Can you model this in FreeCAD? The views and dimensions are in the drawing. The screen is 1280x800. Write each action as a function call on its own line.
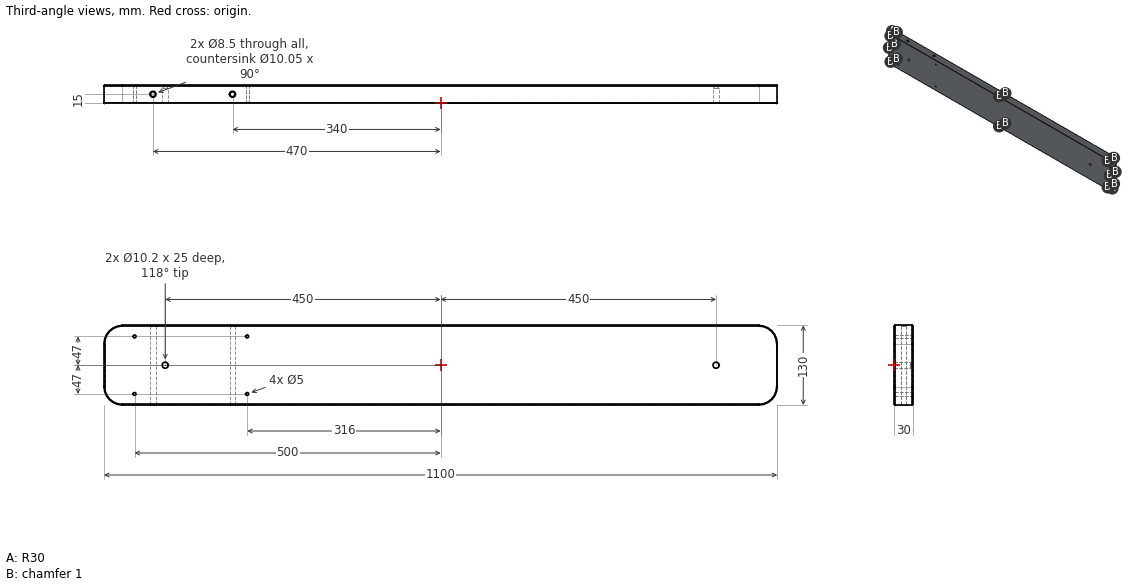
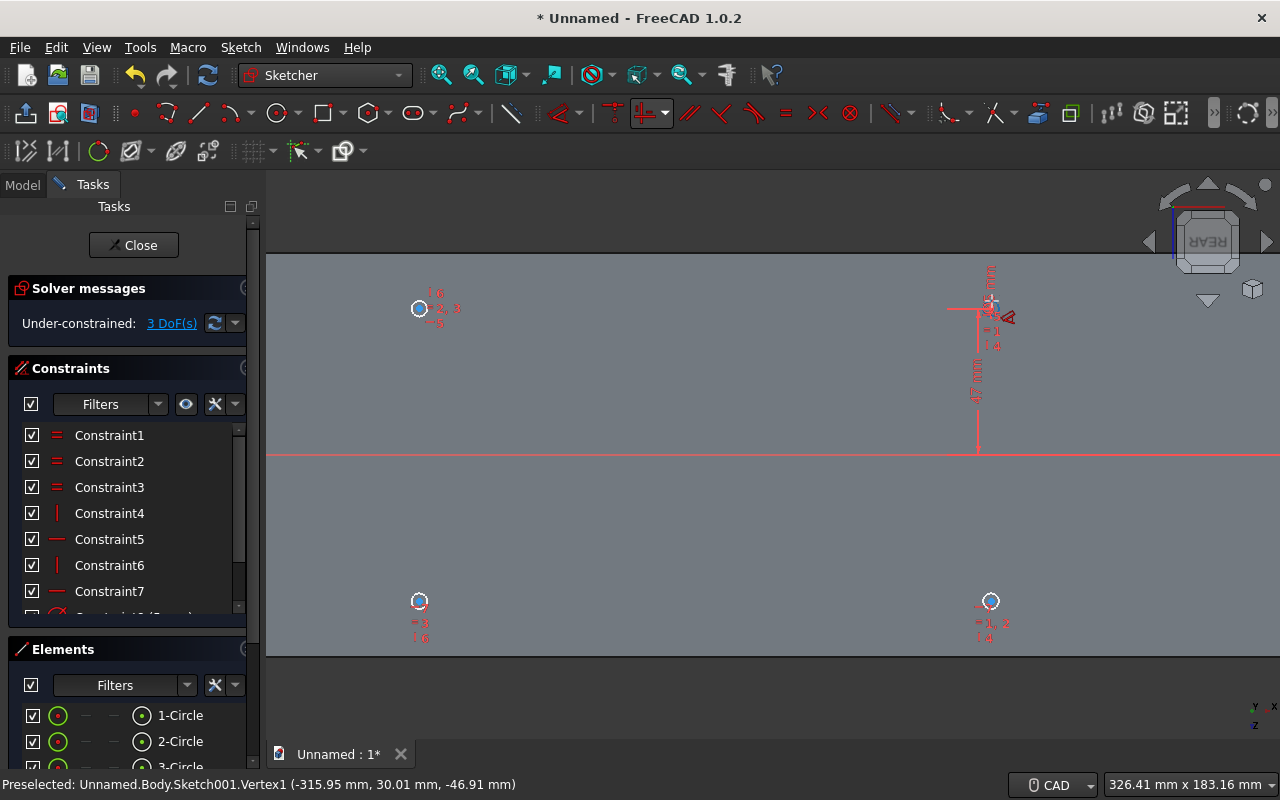
click(991, 601)
click(957, 528)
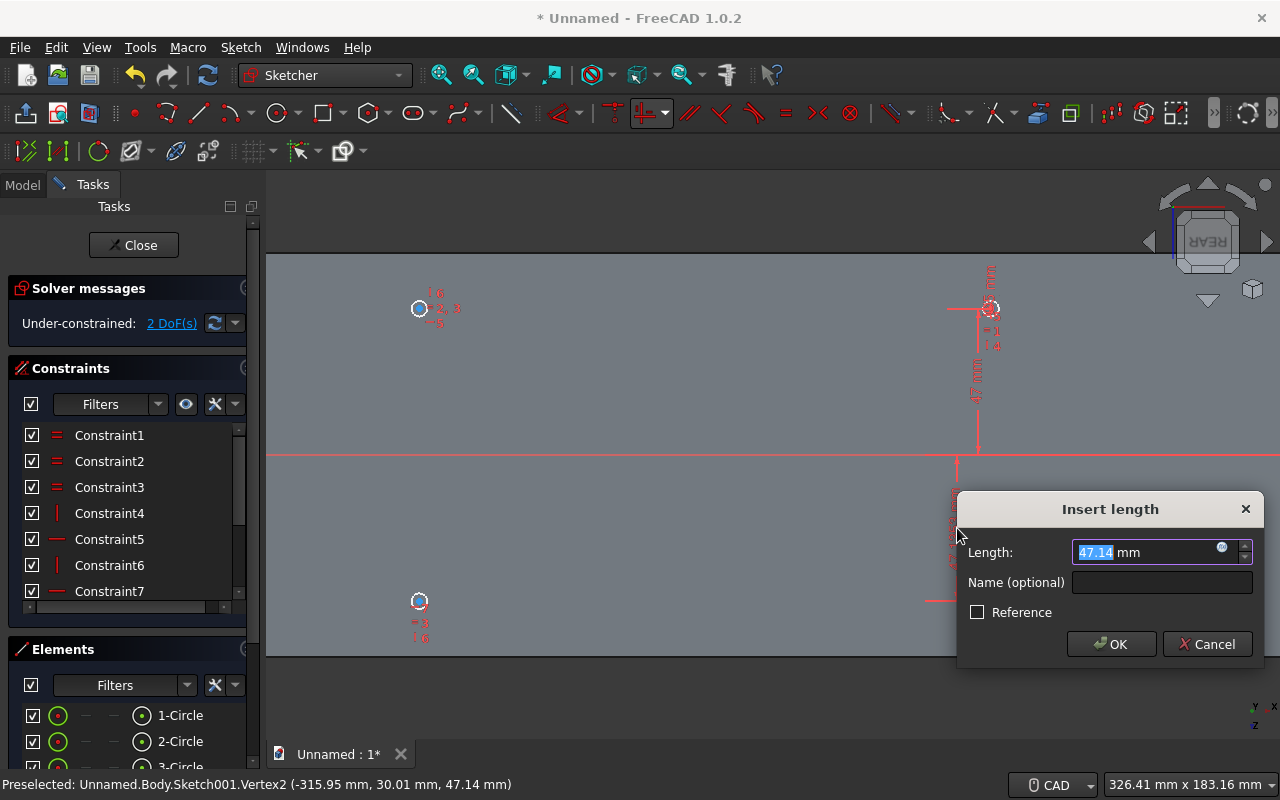
text(47)
key(Return)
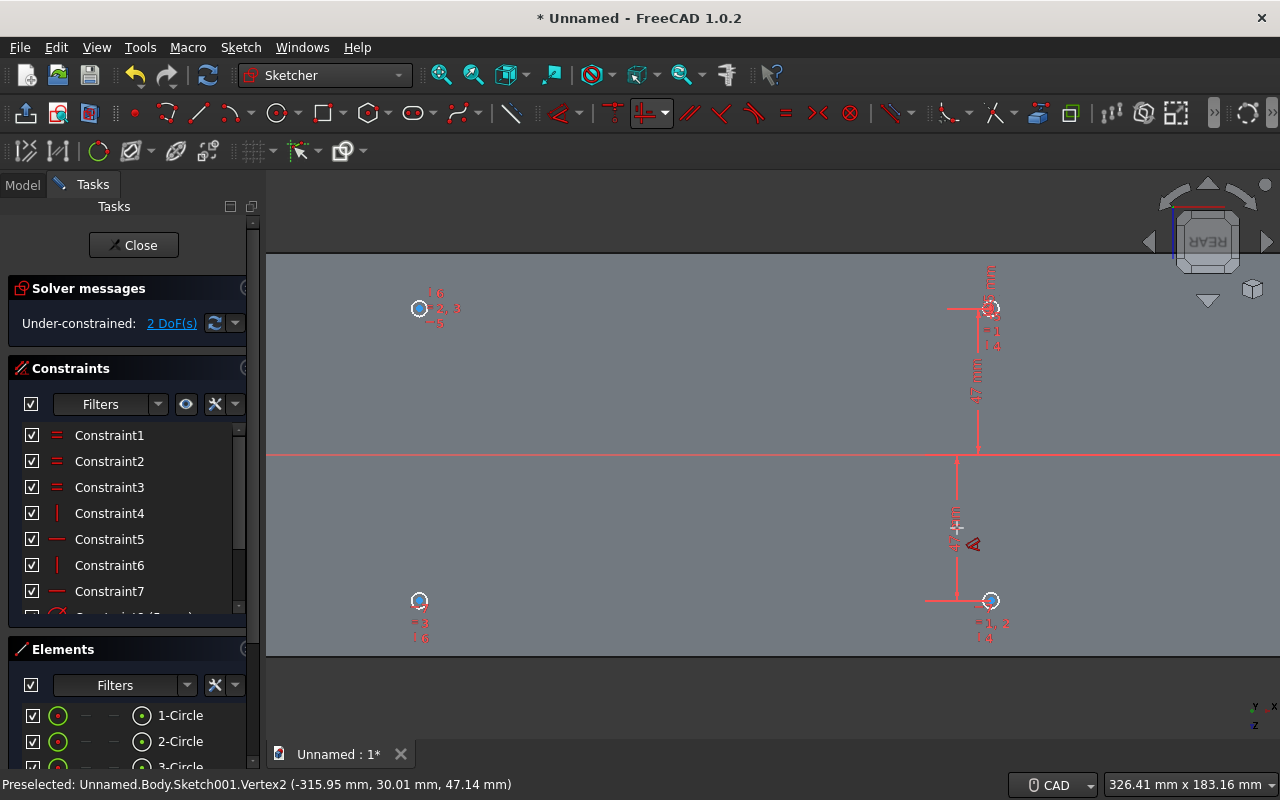
click(991, 309)
click(1082, 275)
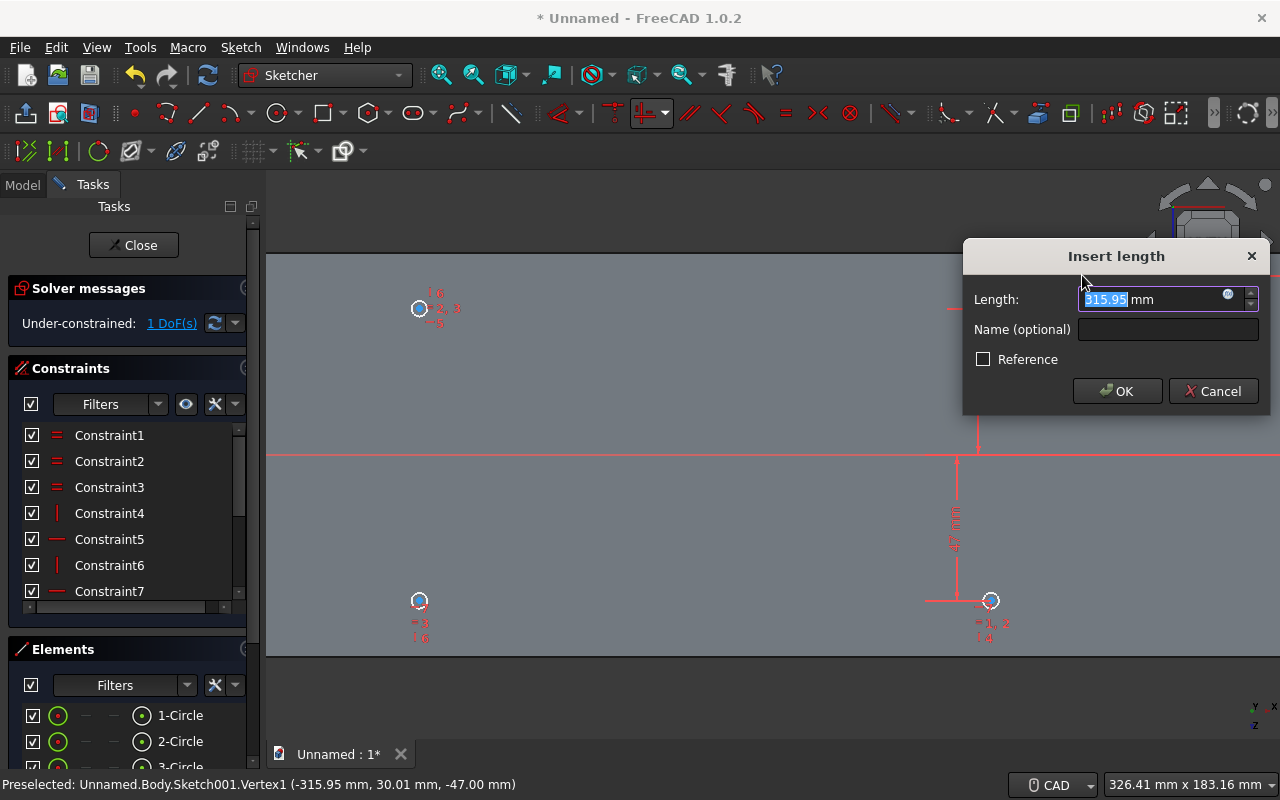
text(316)
key(Return)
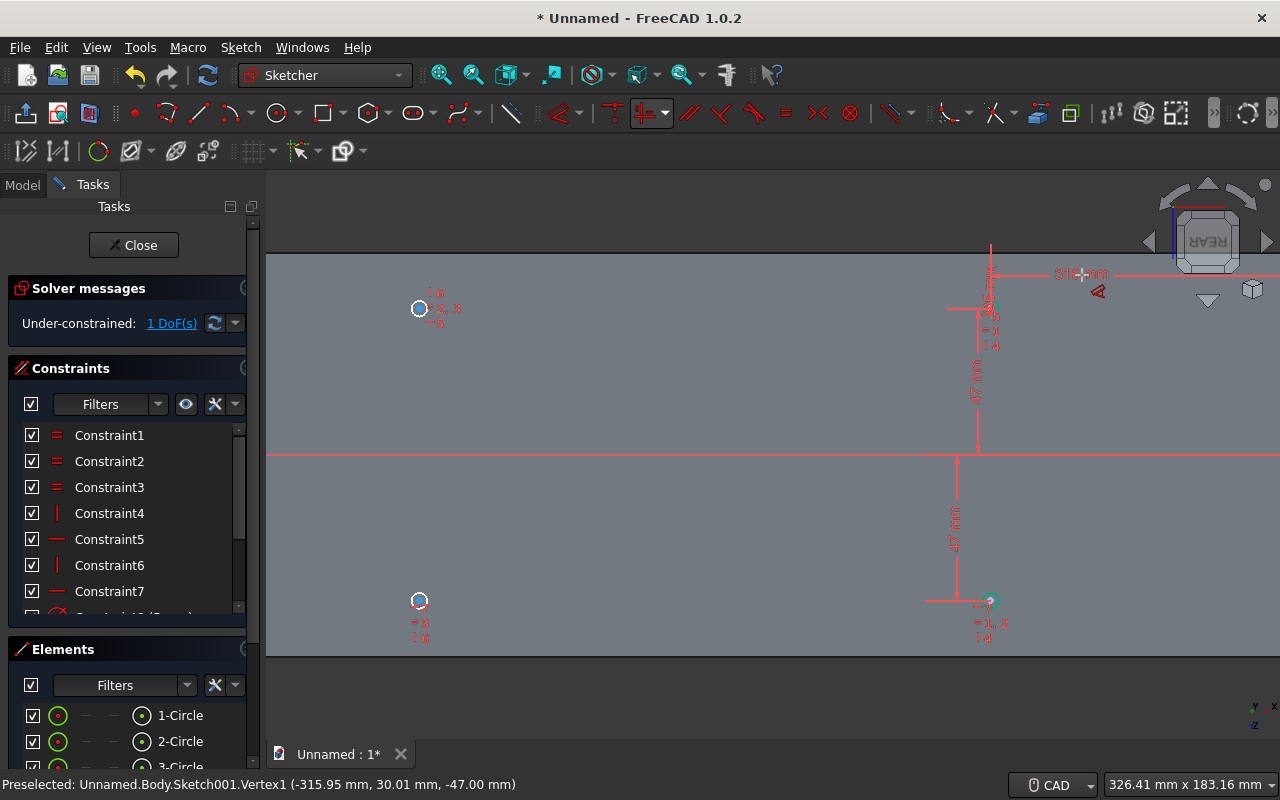
click(419, 309)
click(767, 275)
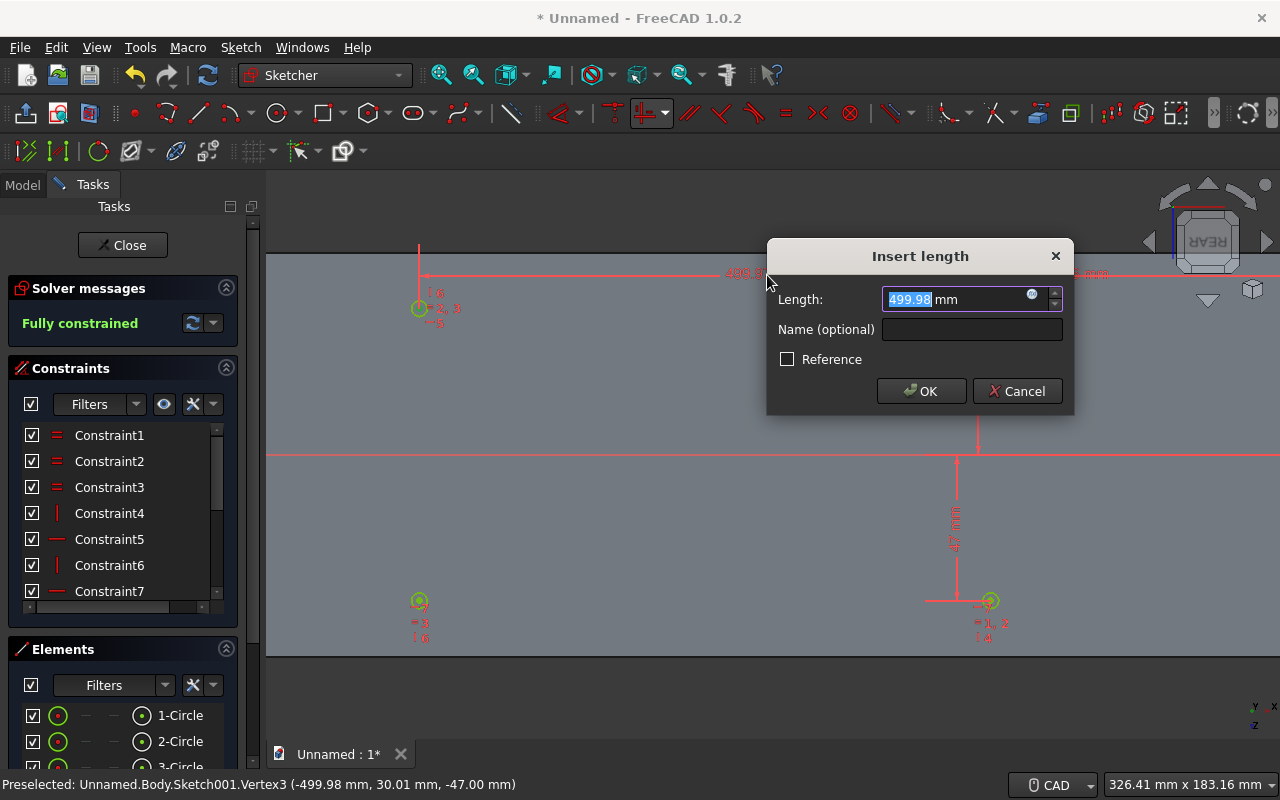
text(500)
key(Return)
key(Escape)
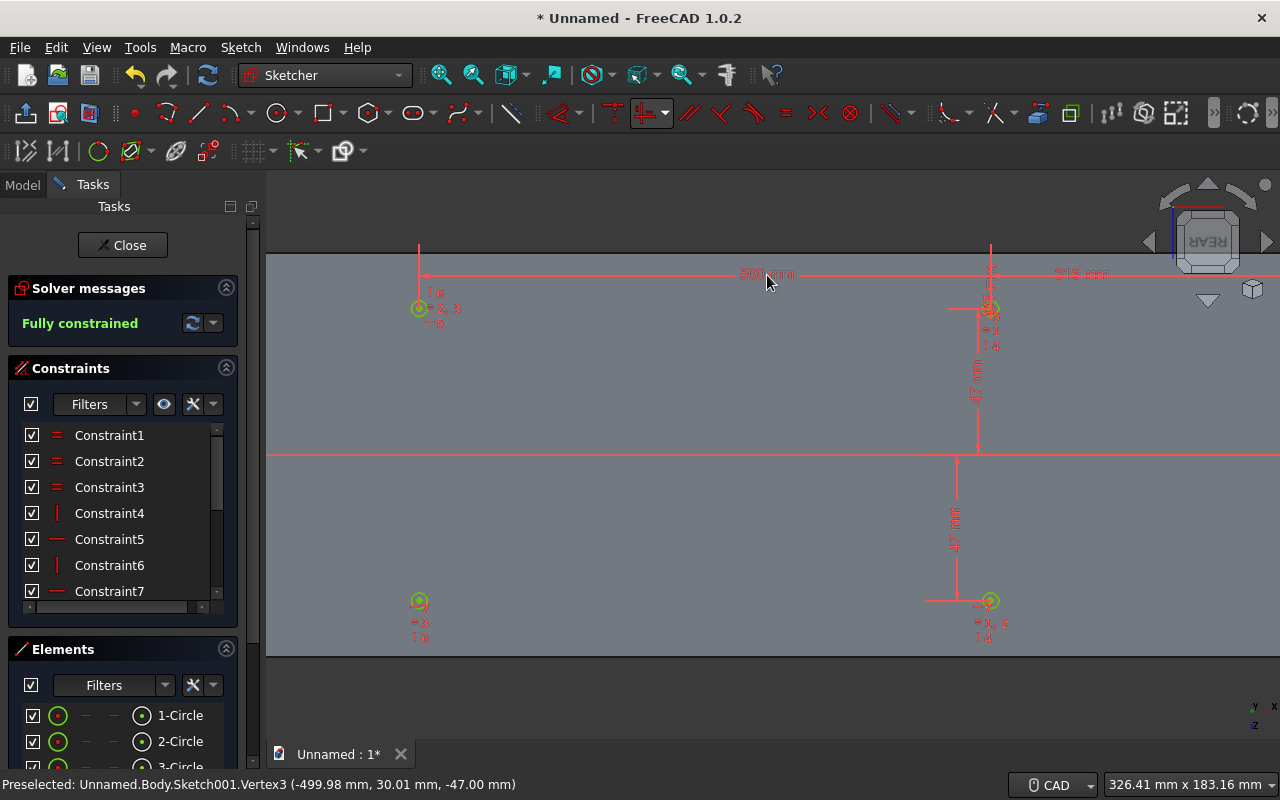
click(123, 245)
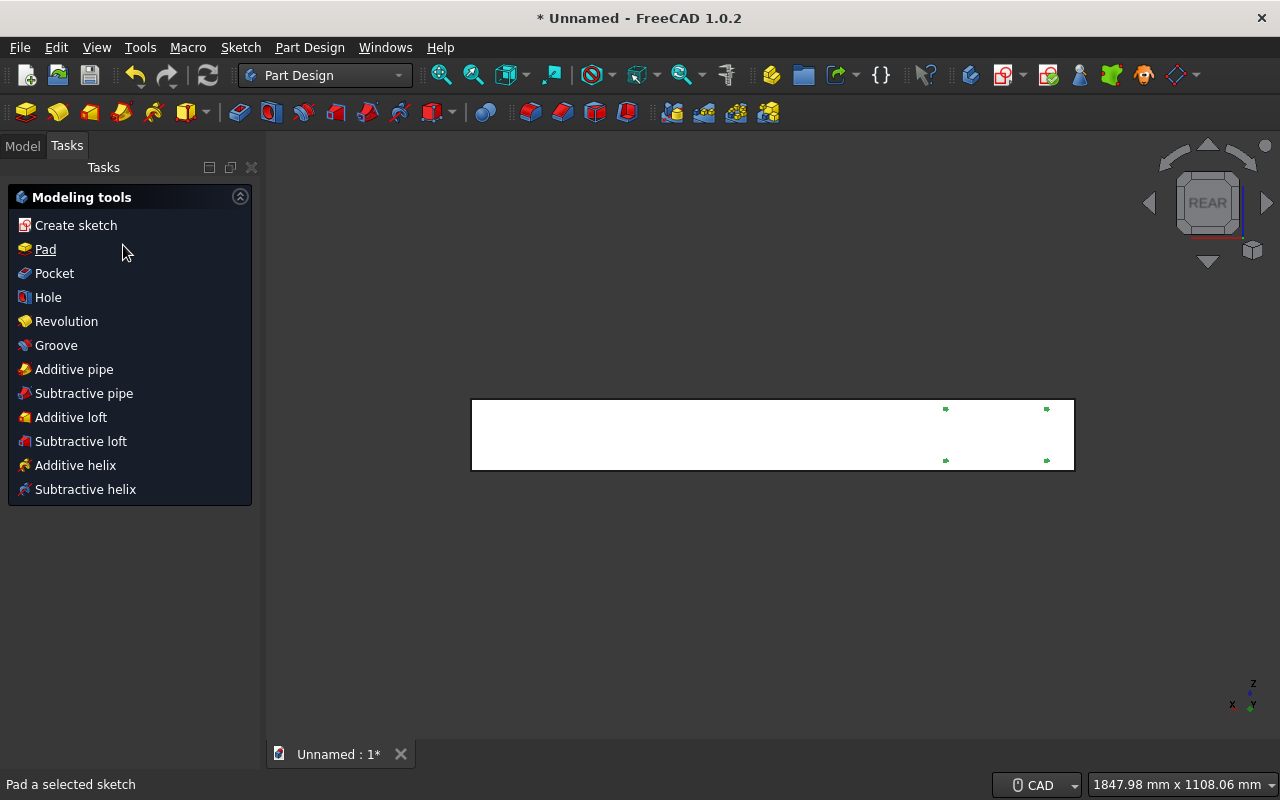
click(240, 112)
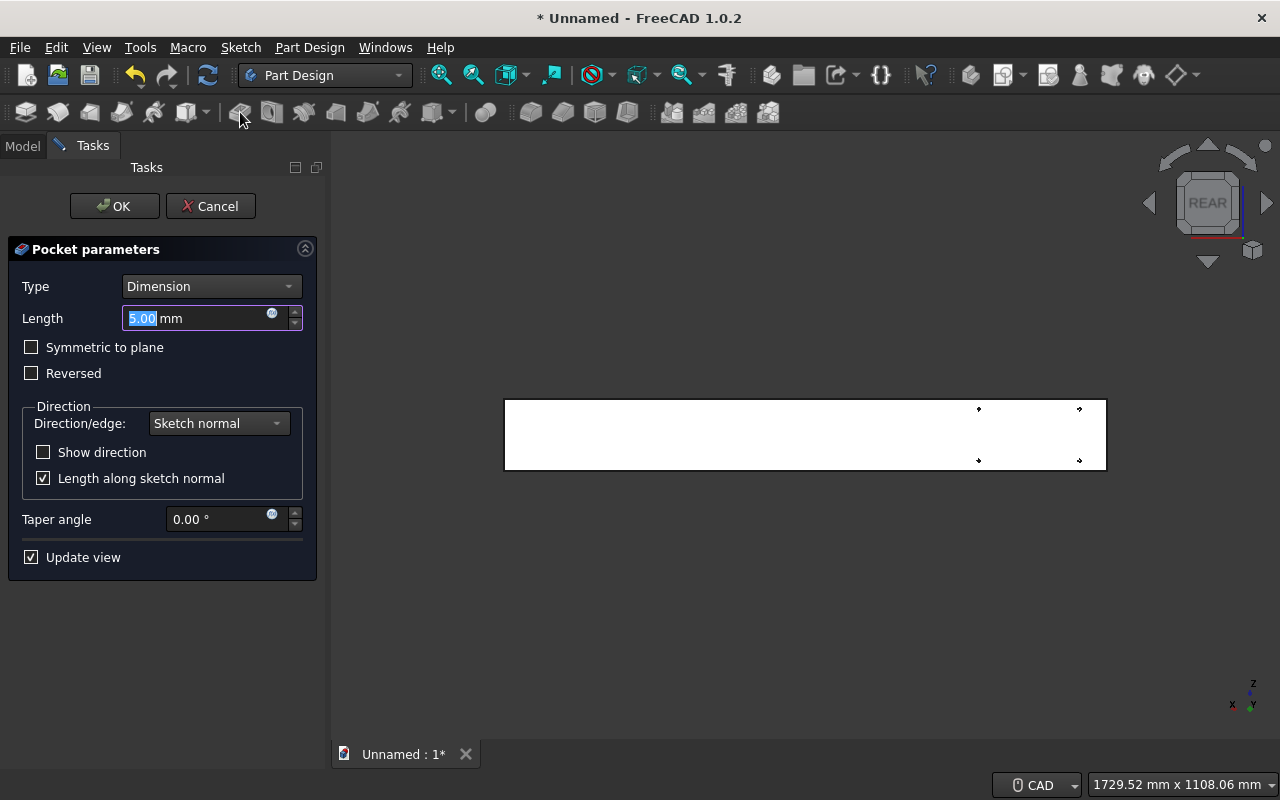
click(212, 286)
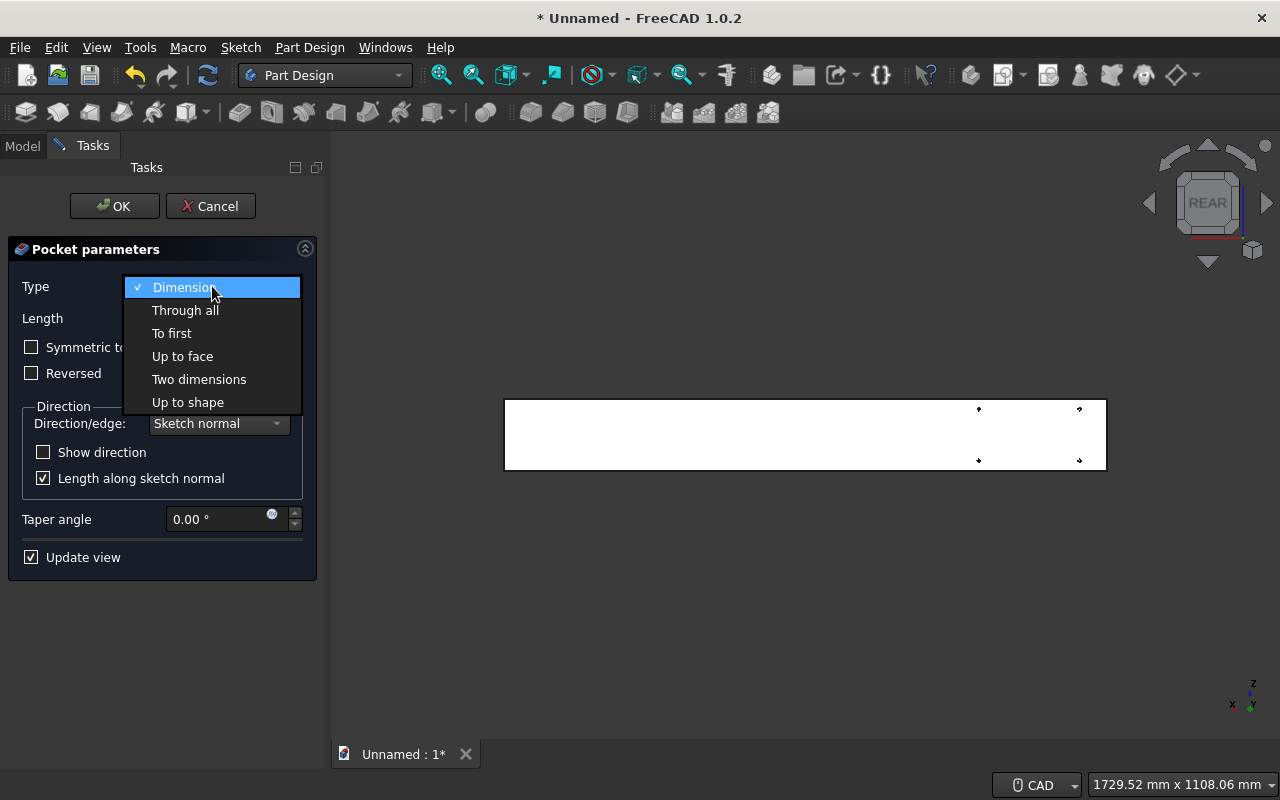
click(212, 310)